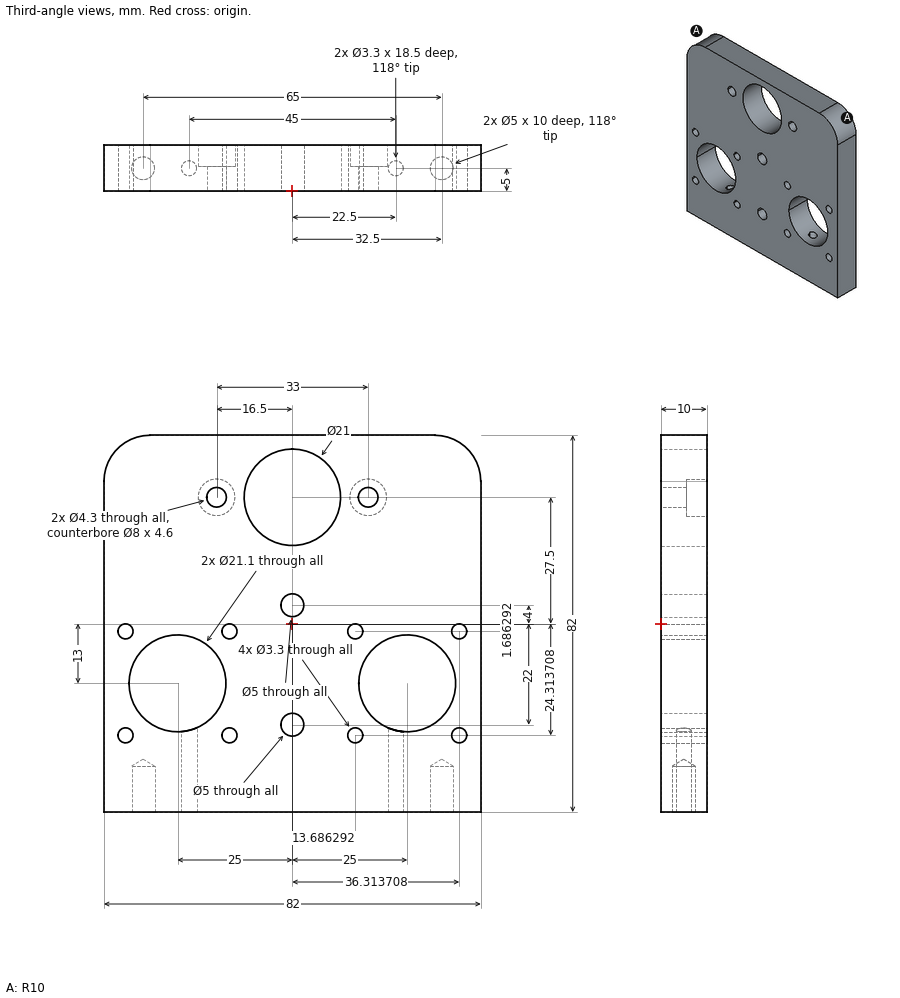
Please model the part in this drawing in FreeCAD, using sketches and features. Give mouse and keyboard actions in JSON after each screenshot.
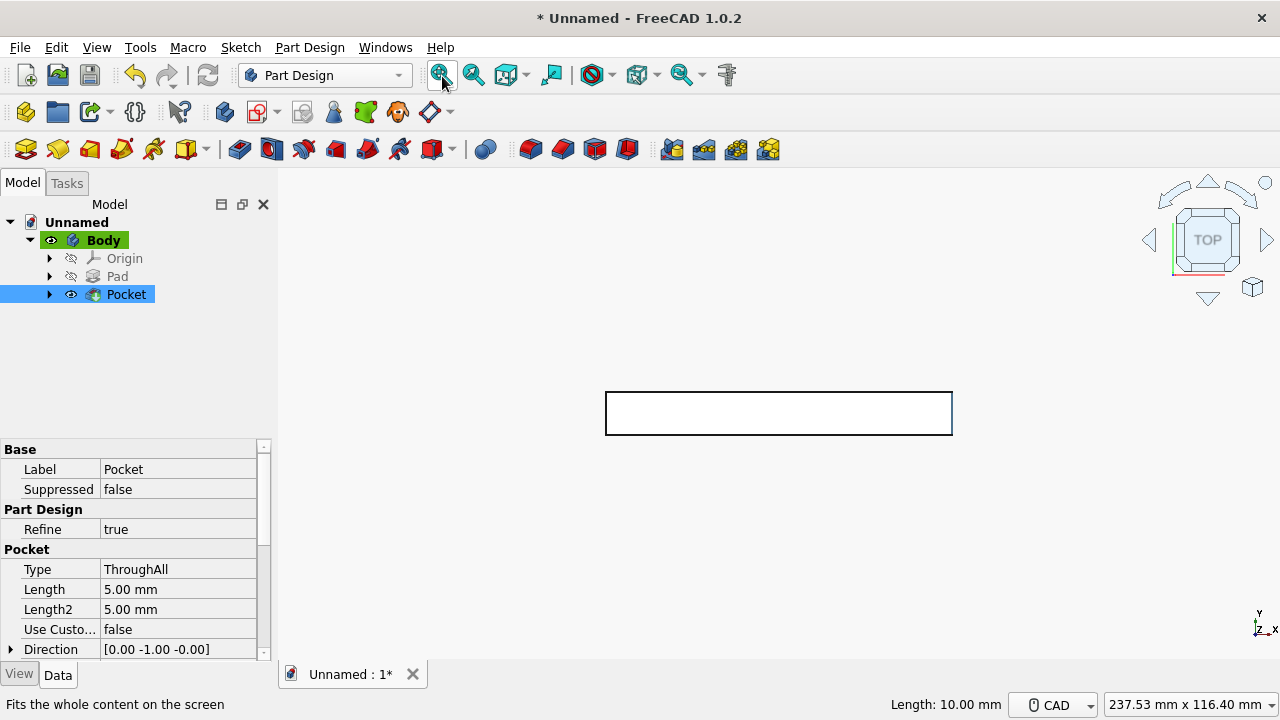
{"action": "left_click", "coordinate": [606, 412], "text": "ctrl"}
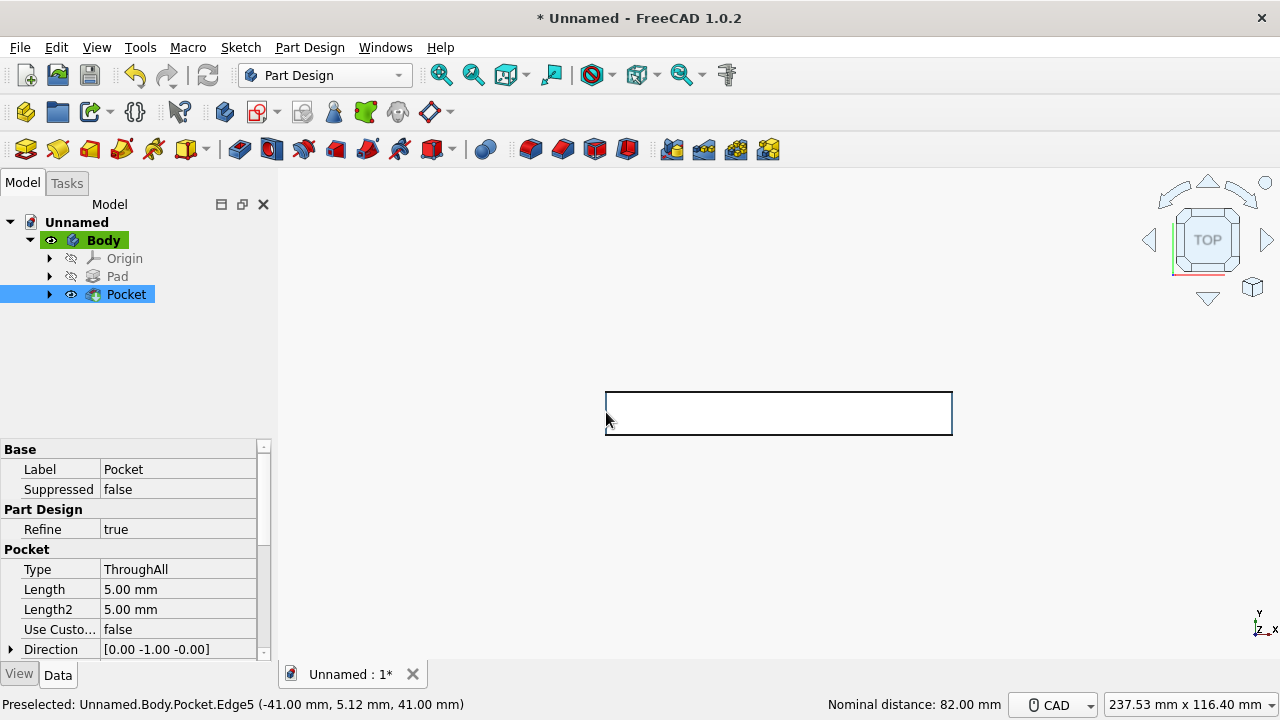
{"action": "left_click", "coordinate": [532, 150]}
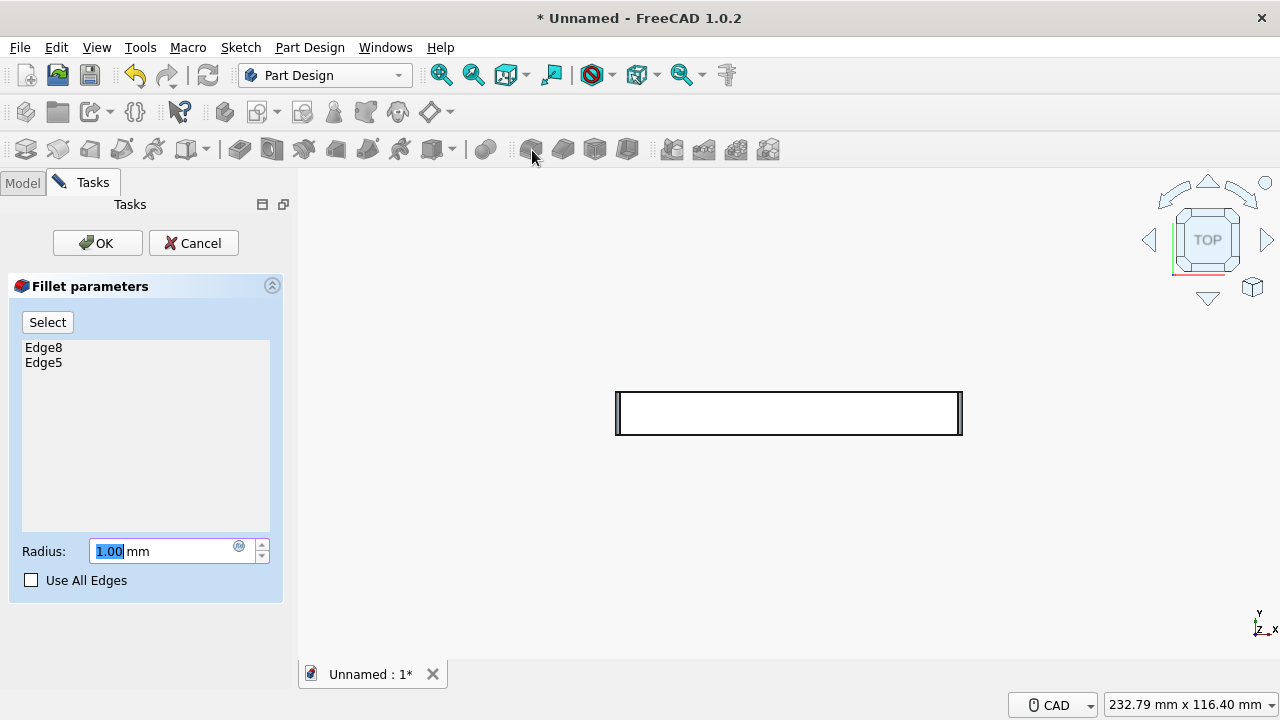
{"action": "type", "text": "10"}
{"action": "key", "text": "Tab"}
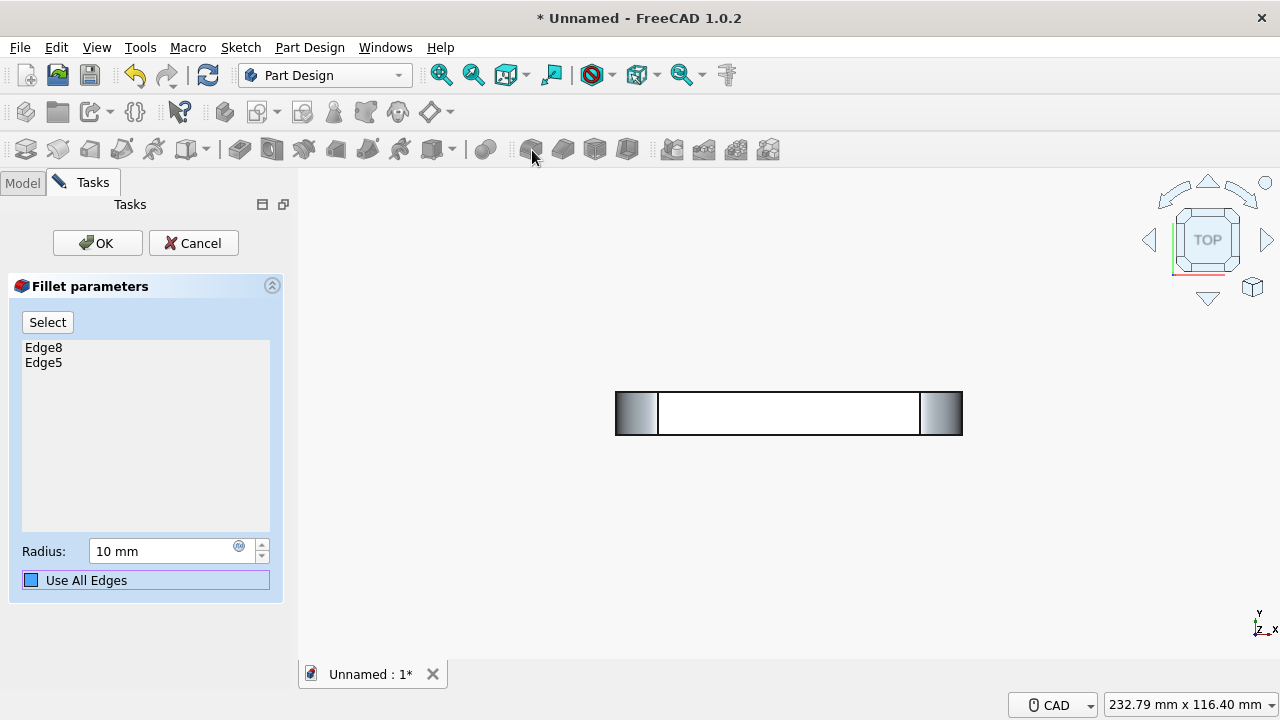
{"action": "left_click", "coordinate": [98, 243]}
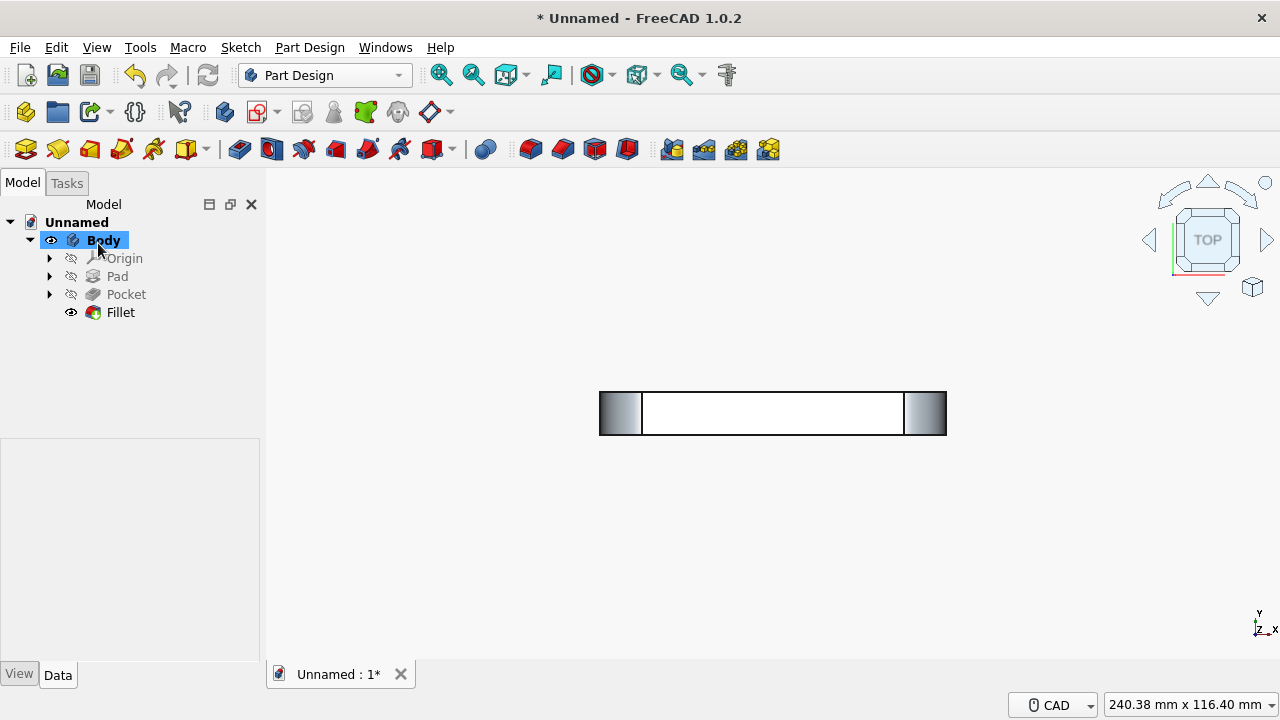
{"action": "left_click", "coordinate": [442, 76]}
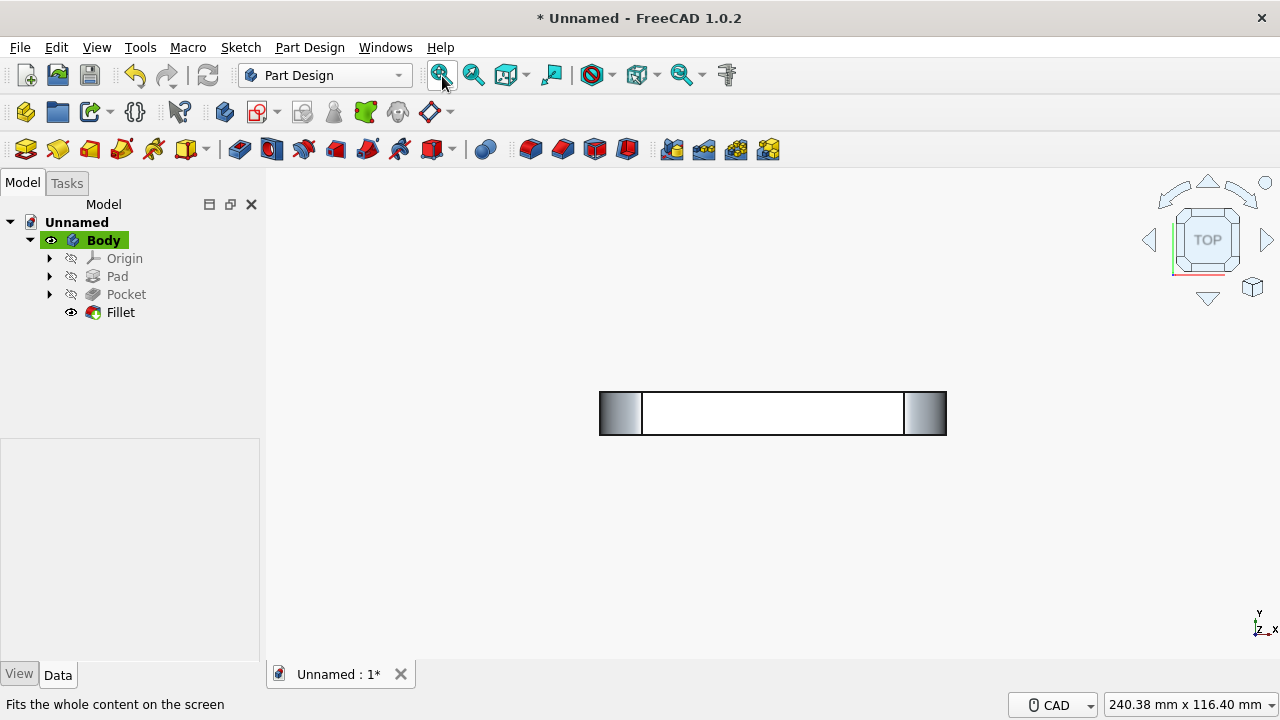
{"action": "key", "text": "4"}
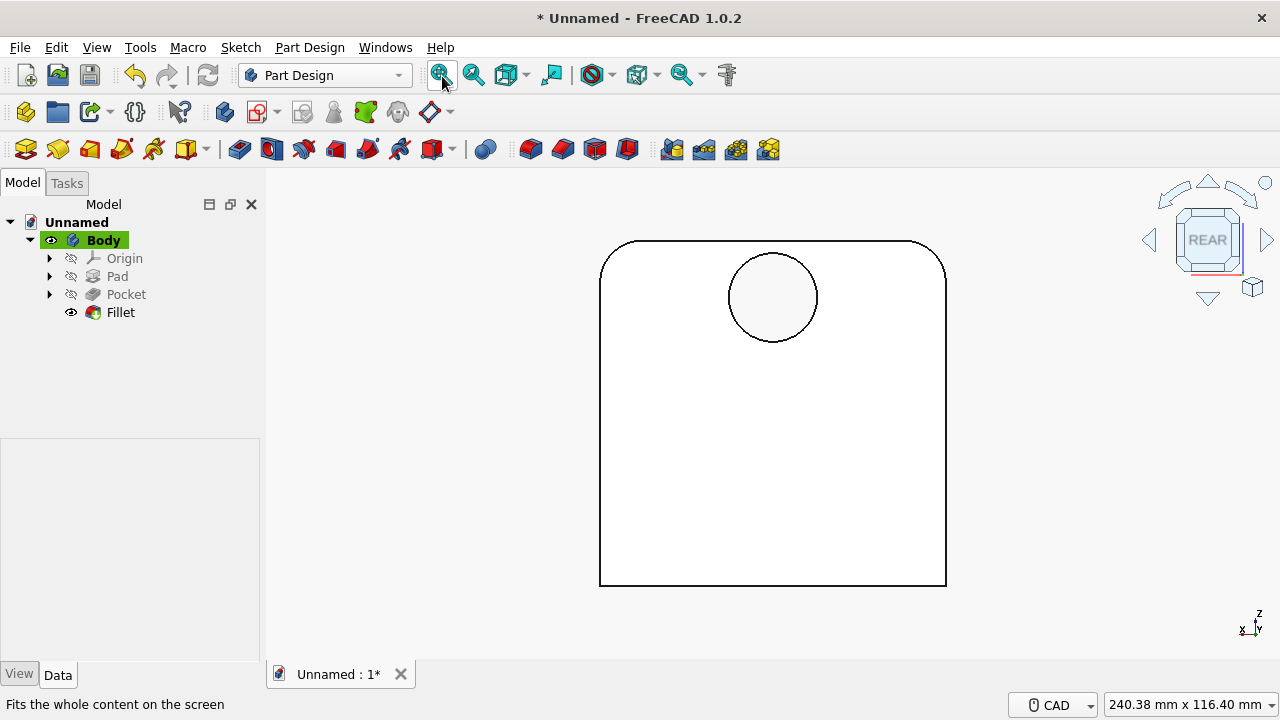
{"action": "left_click", "coordinate": [724, 462]}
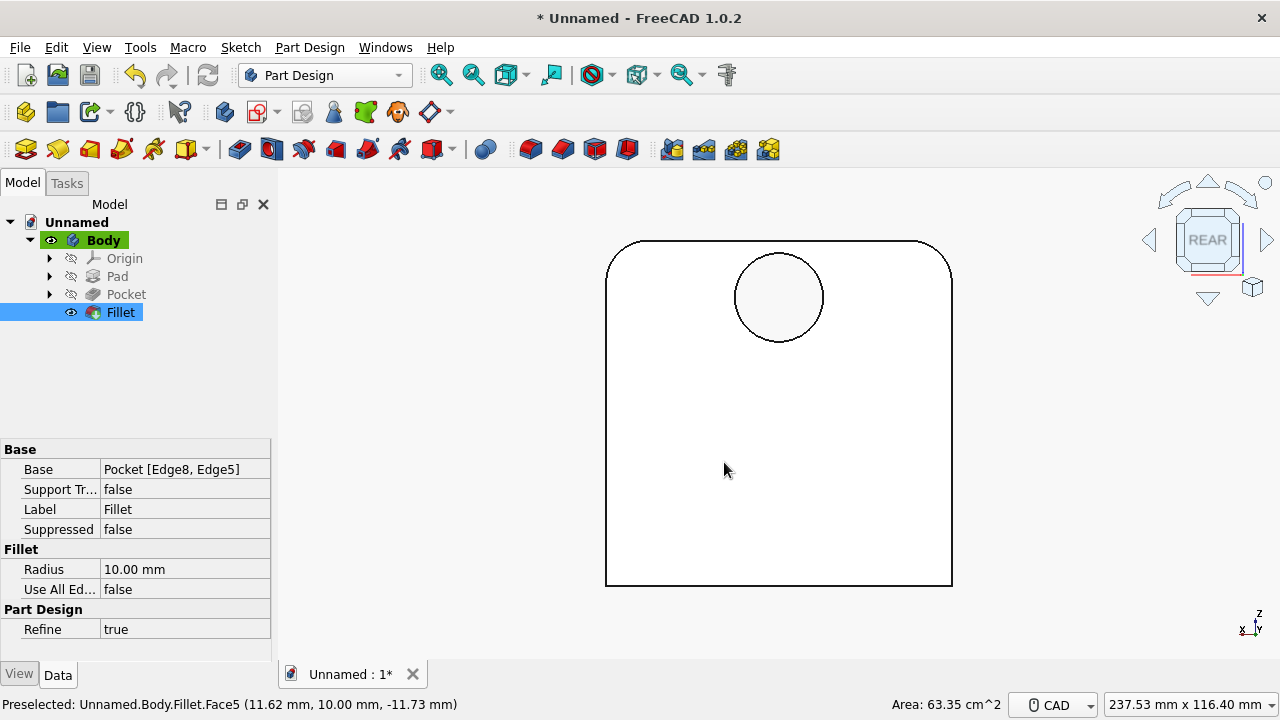
{"action": "left_click", "coordinate": [258, 112]}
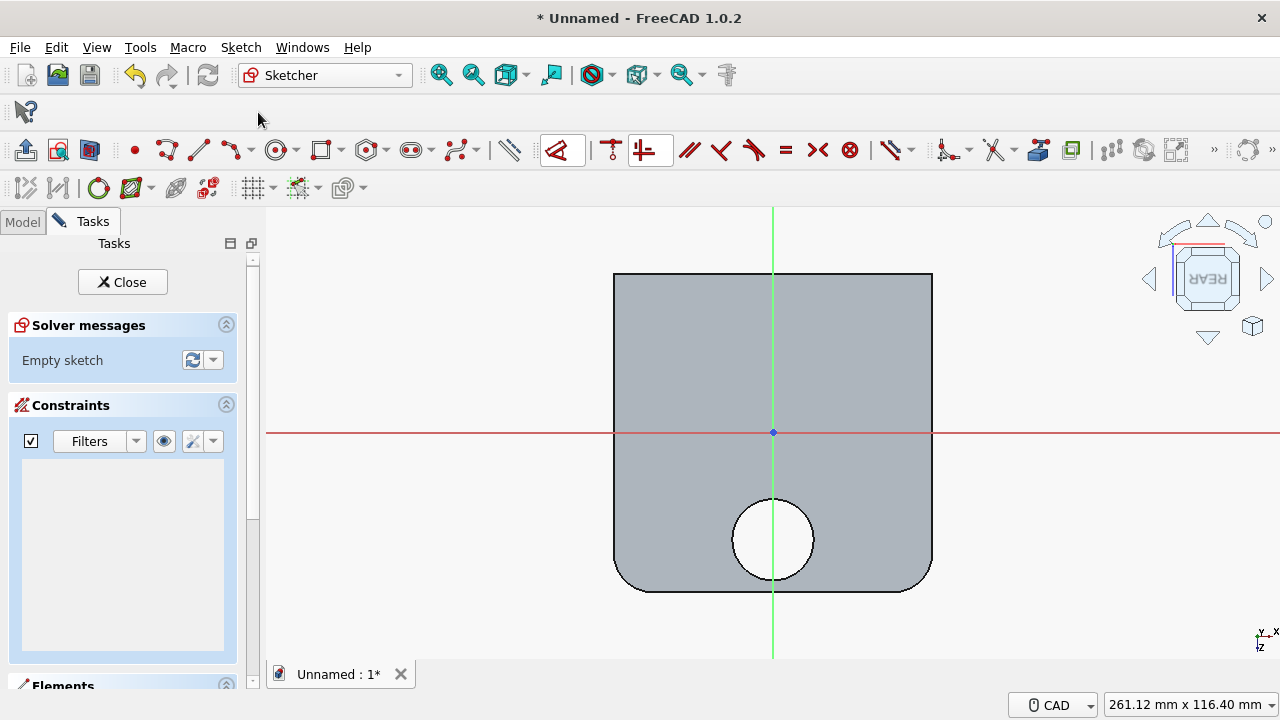
{"action": "scroll", "coordinate": [829, 538], "scroll_direction": "up", "scroll_amount": 4}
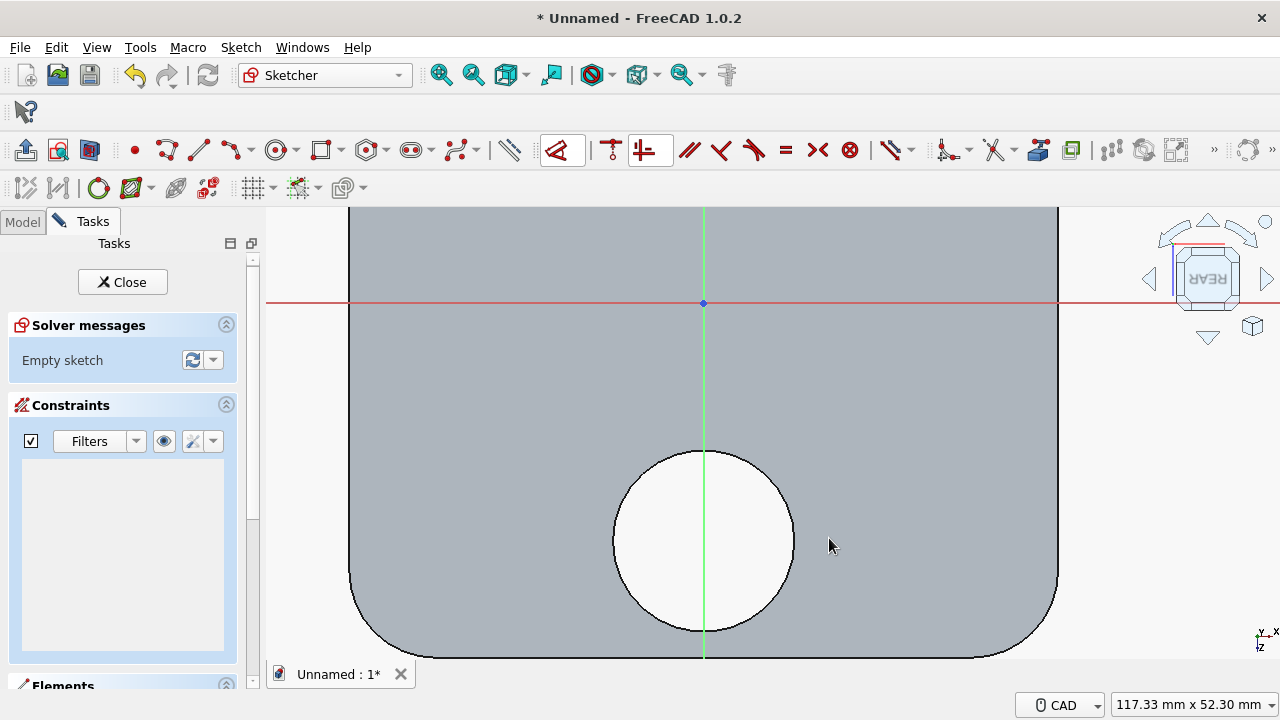
{"action": "left_click", "coordinate": [276, 150]}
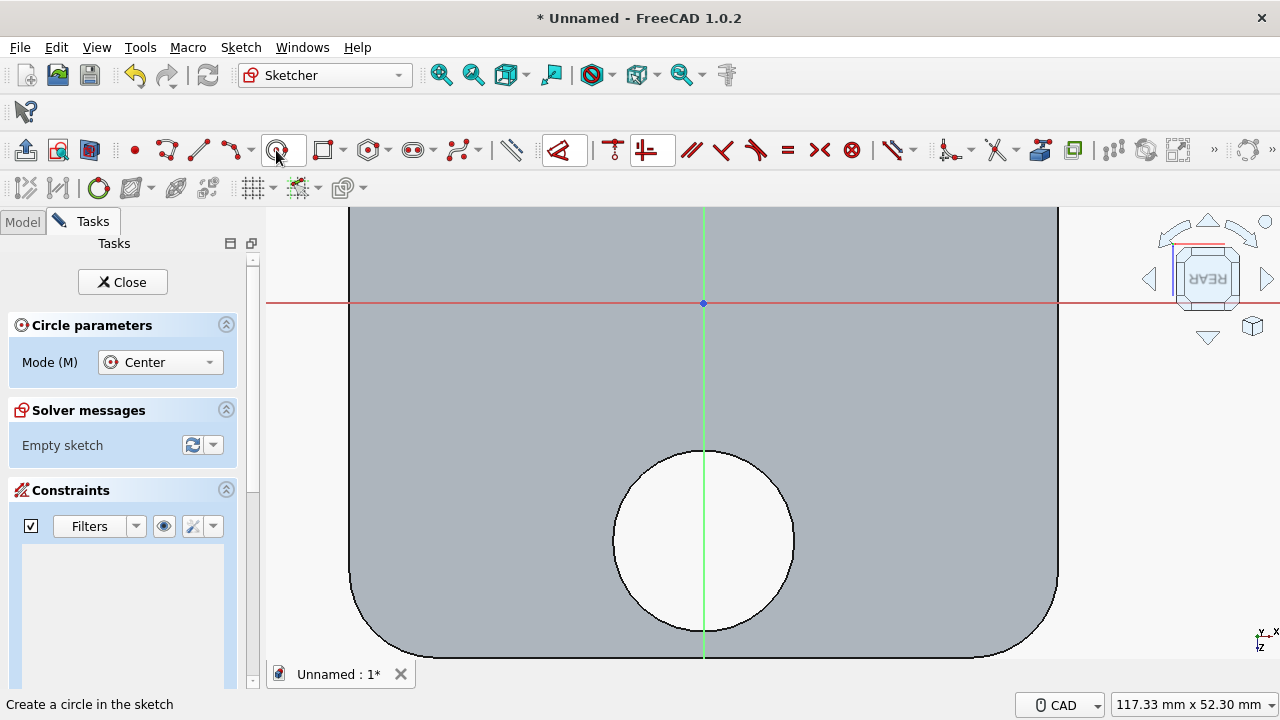
{"action": "left_click", "coordinate": [561, 541]}
{"action": "left_click", "coordinate": [574, 528]}